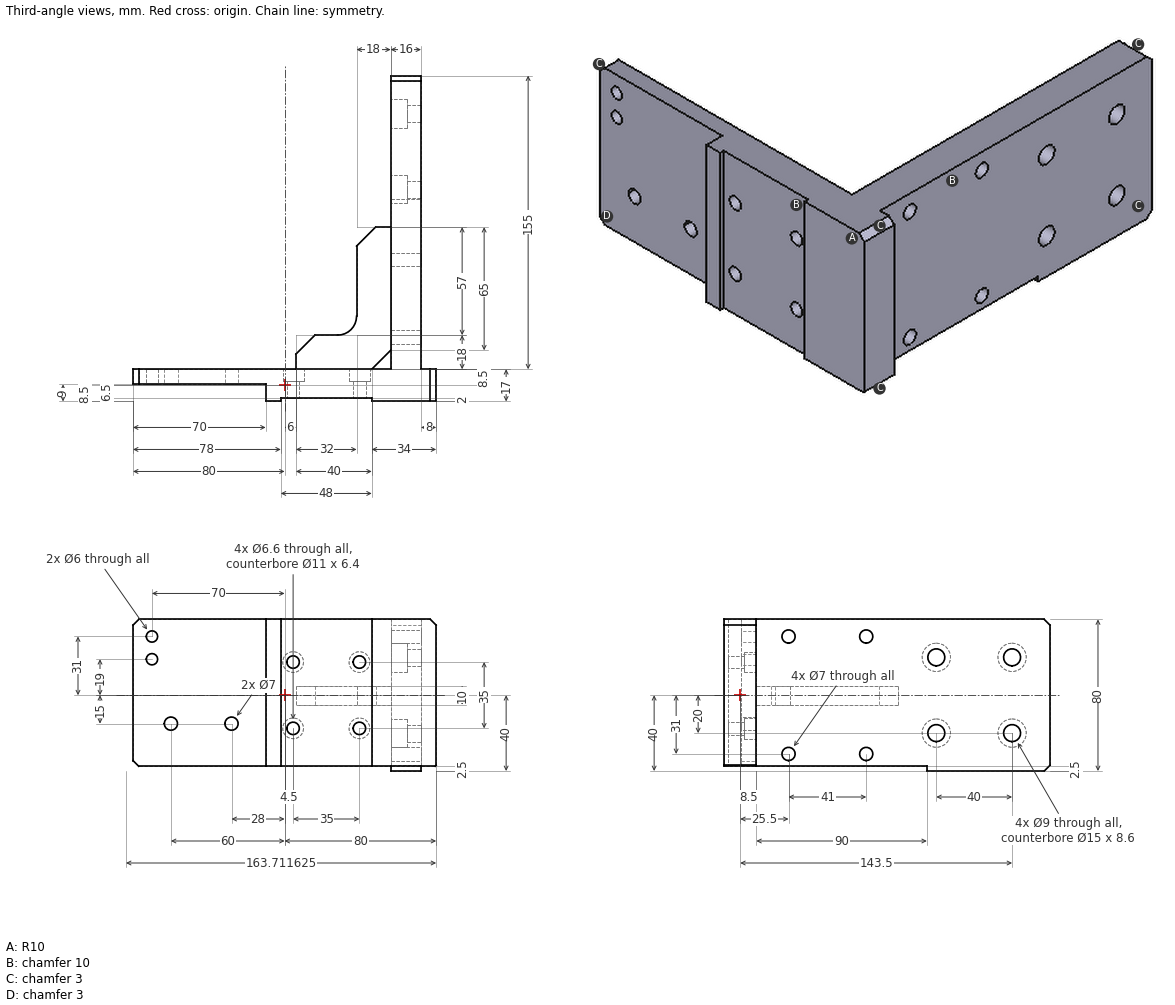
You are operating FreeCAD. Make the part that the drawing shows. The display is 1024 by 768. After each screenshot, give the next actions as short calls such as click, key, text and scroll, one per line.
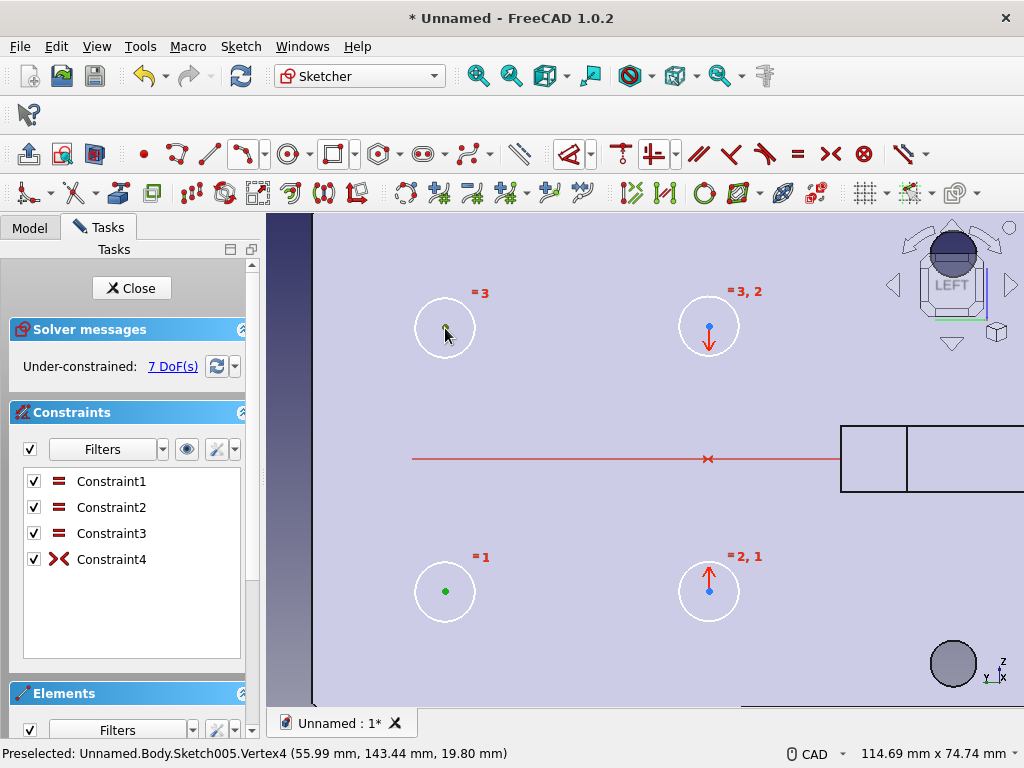
click(415, 459)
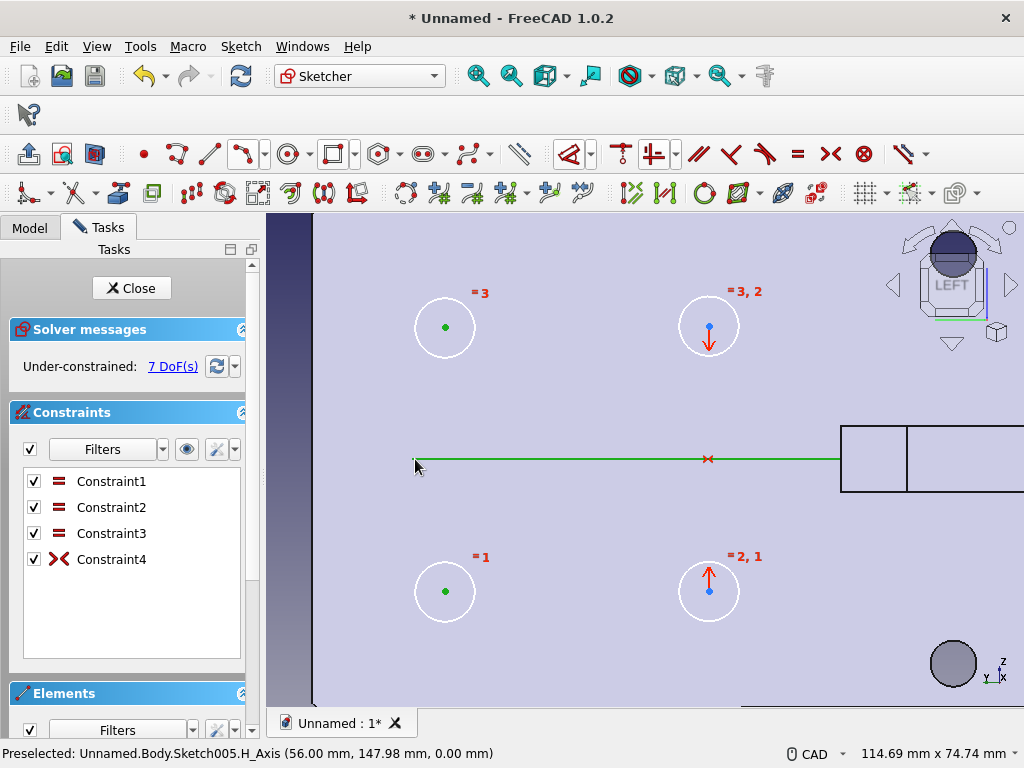
click(831, 154)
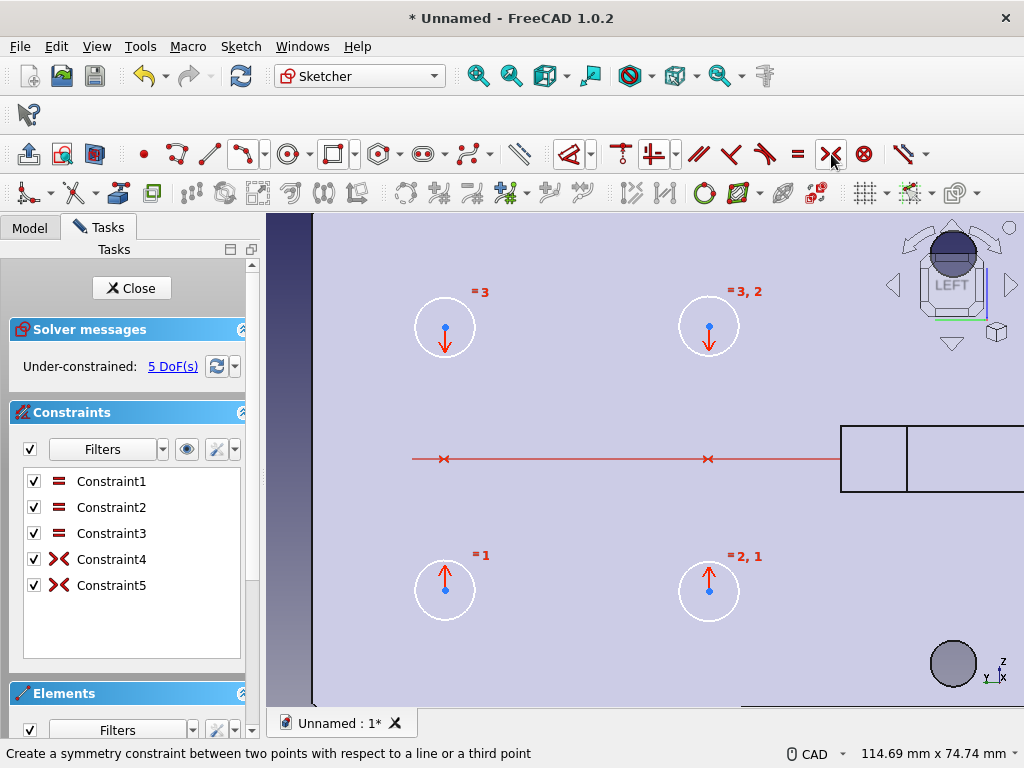
click(466, 569)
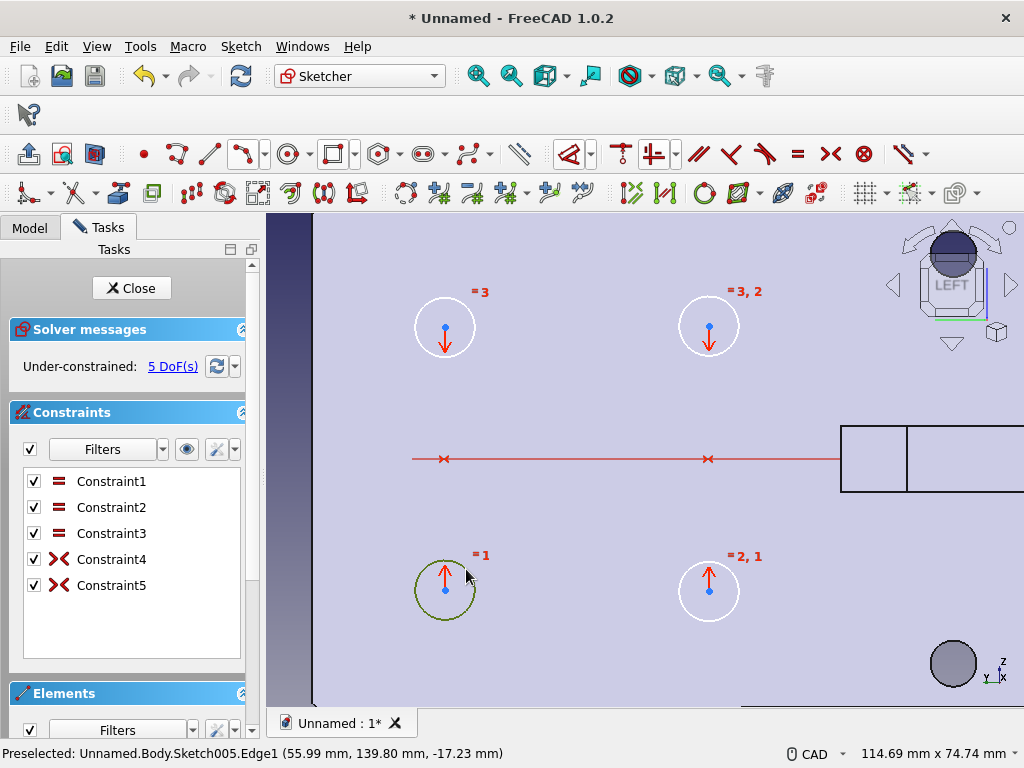
key(k)
key(o)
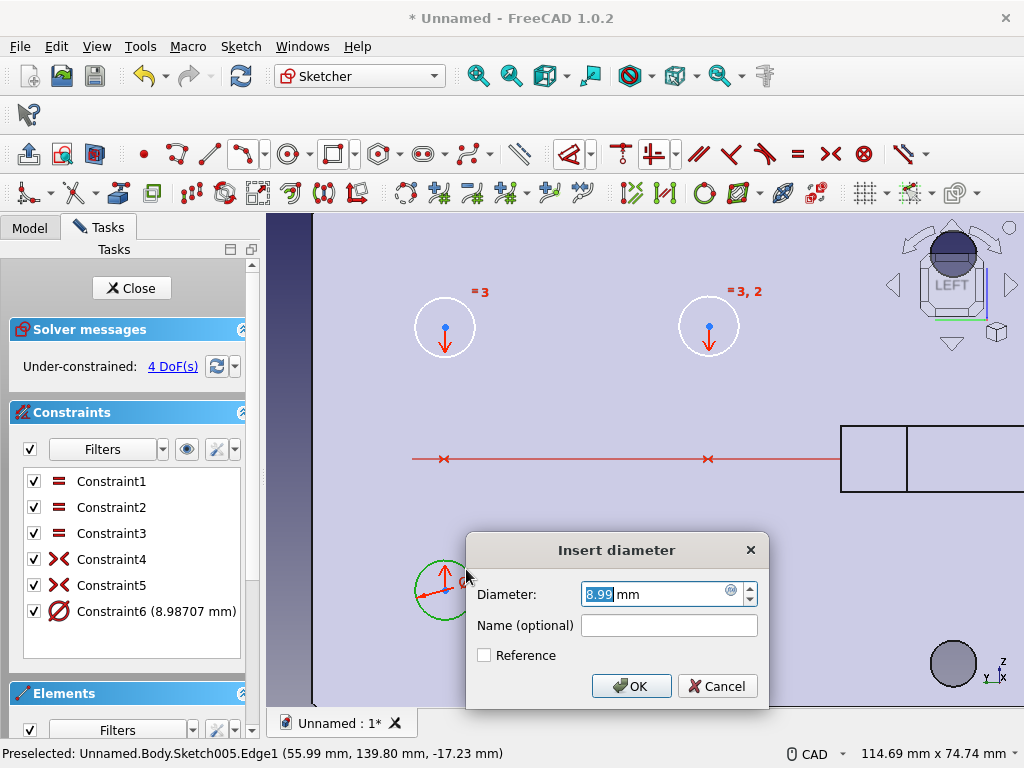
text(9)
key(Return)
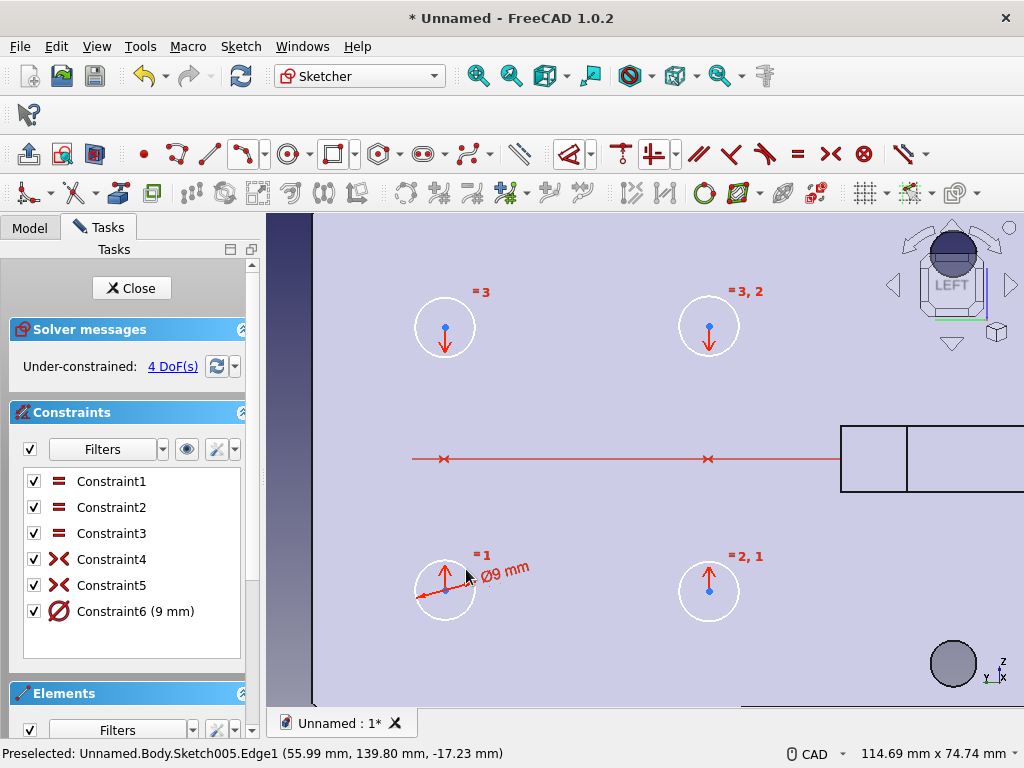
click(445, 590)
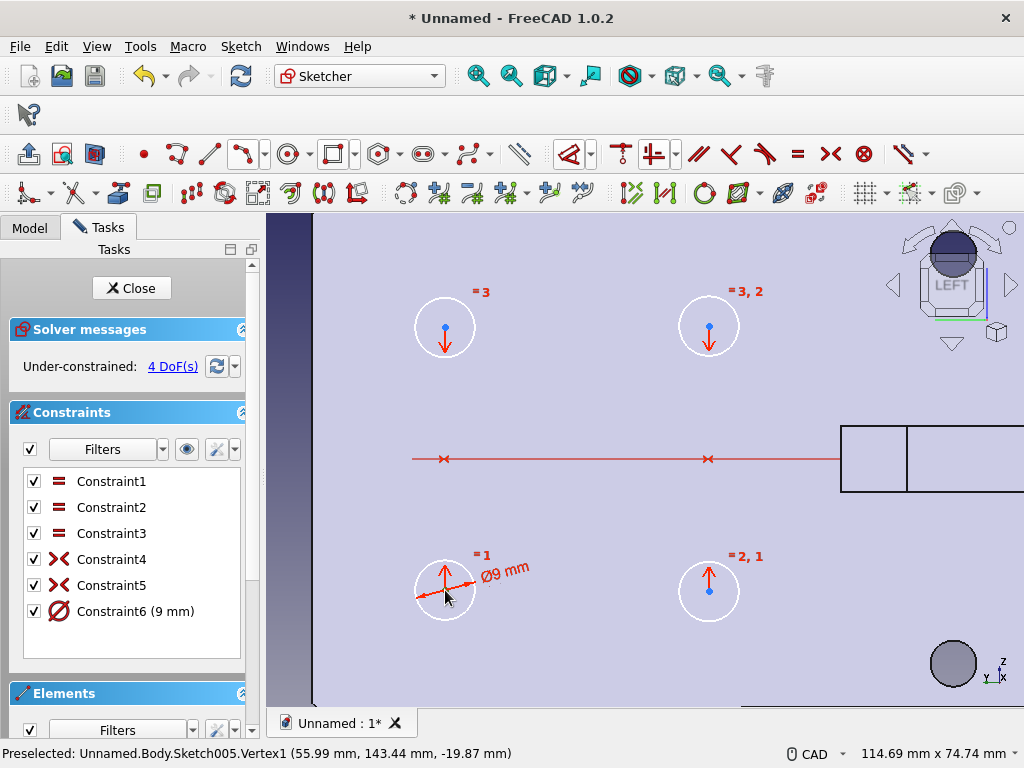
click(590, 154)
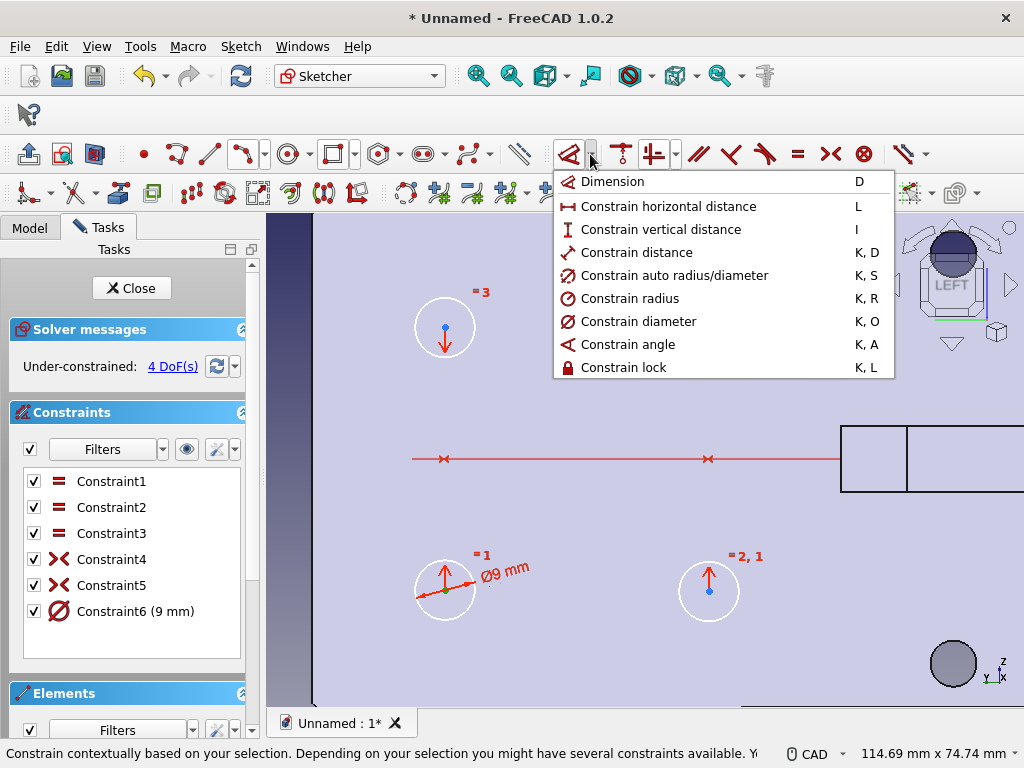
click(724, 230)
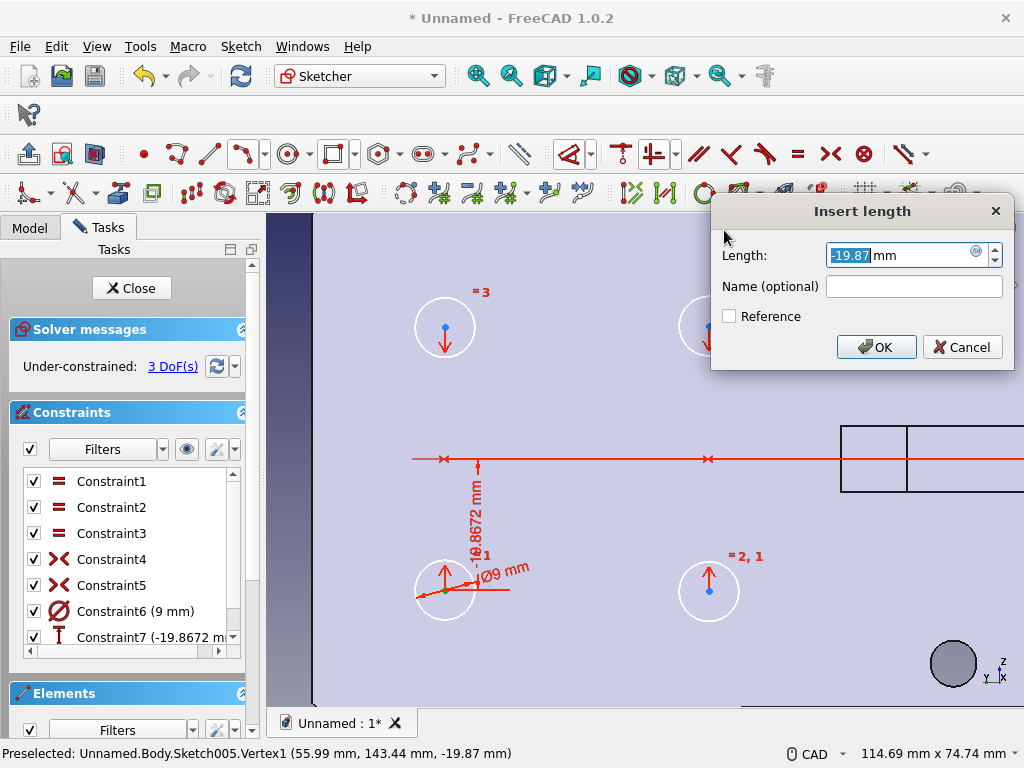
text(-20)
key(Return)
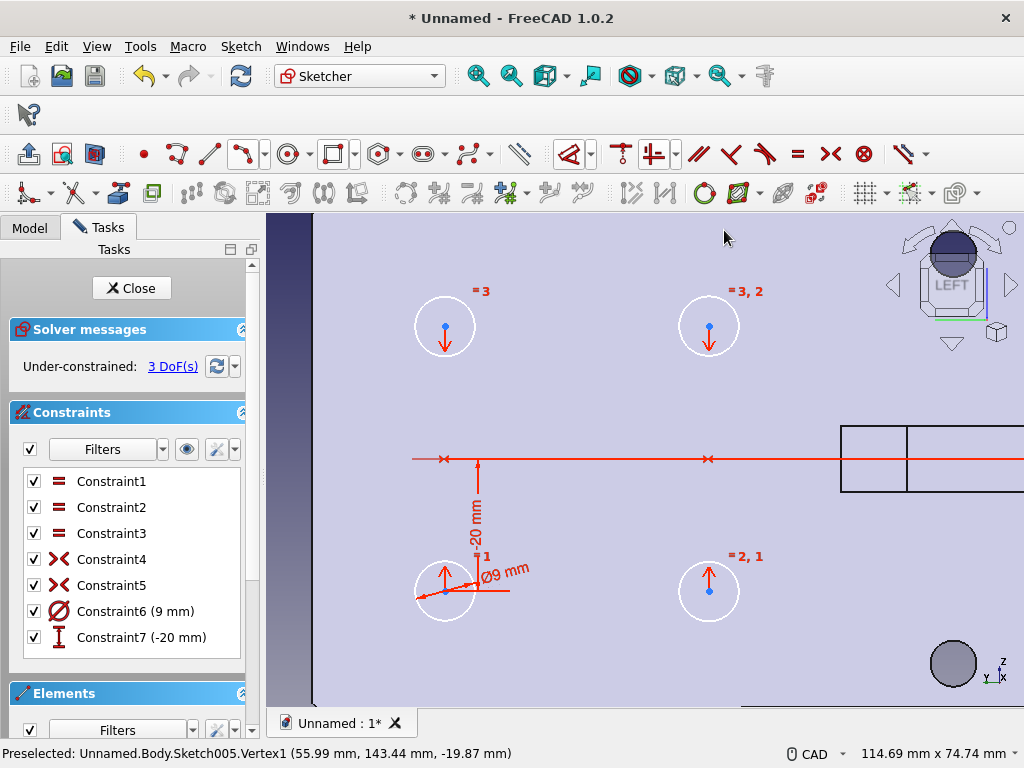
click(709, 592)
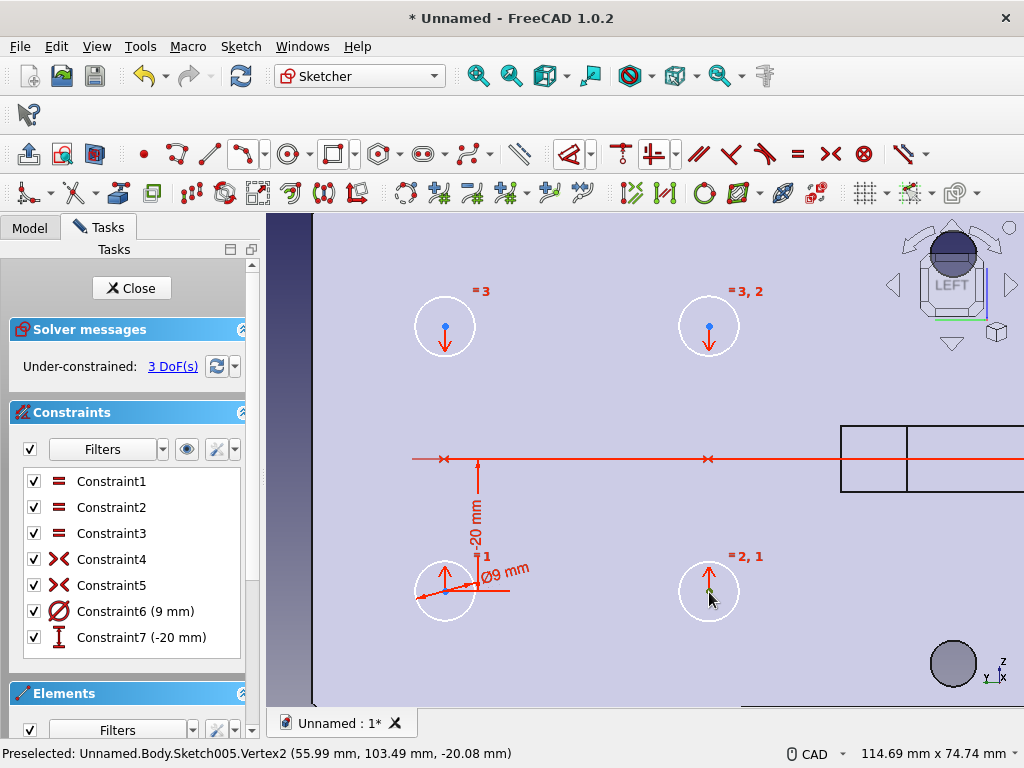
click(590, 154)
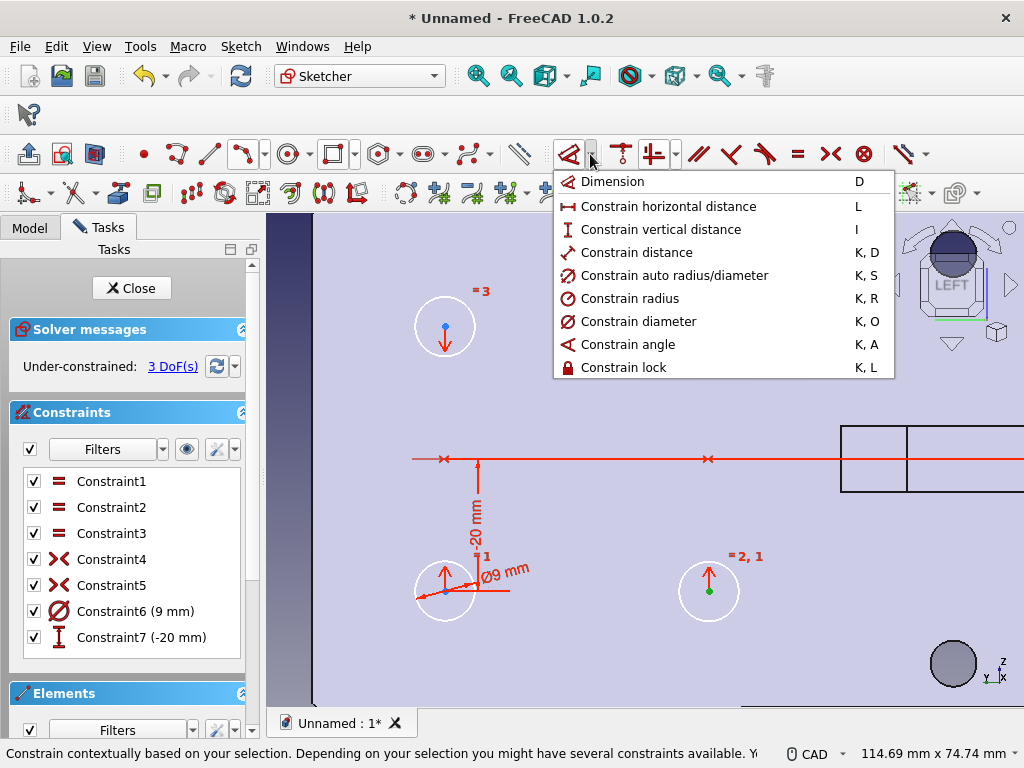
click(724, 230)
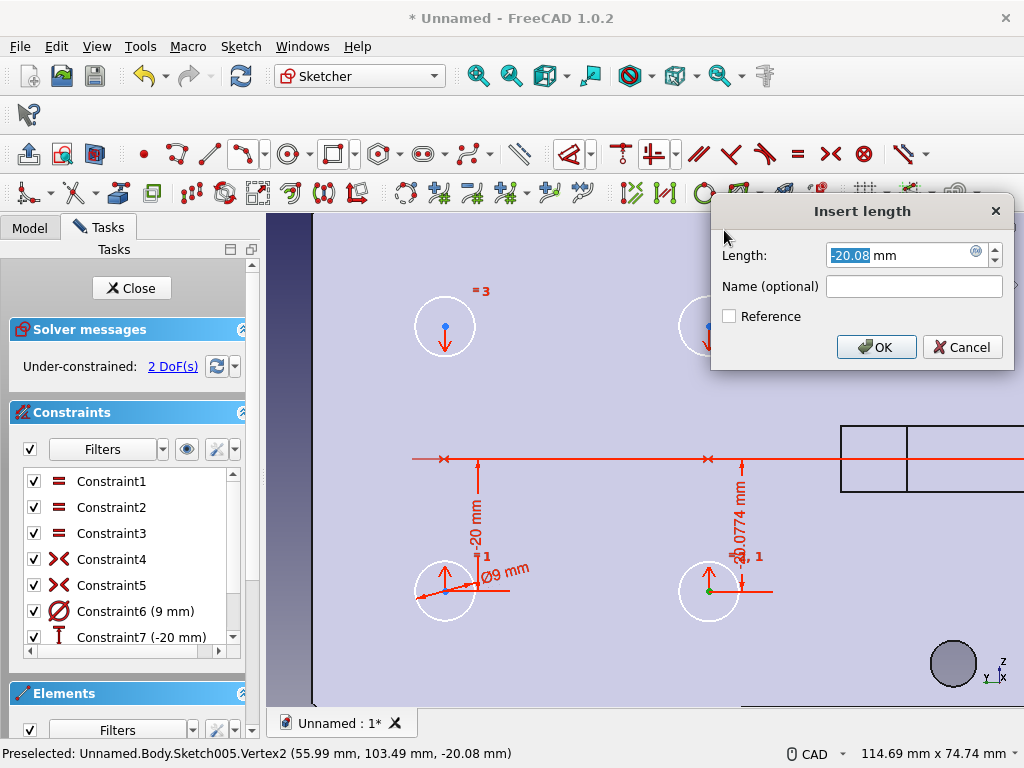
text(-20)
key(Return)